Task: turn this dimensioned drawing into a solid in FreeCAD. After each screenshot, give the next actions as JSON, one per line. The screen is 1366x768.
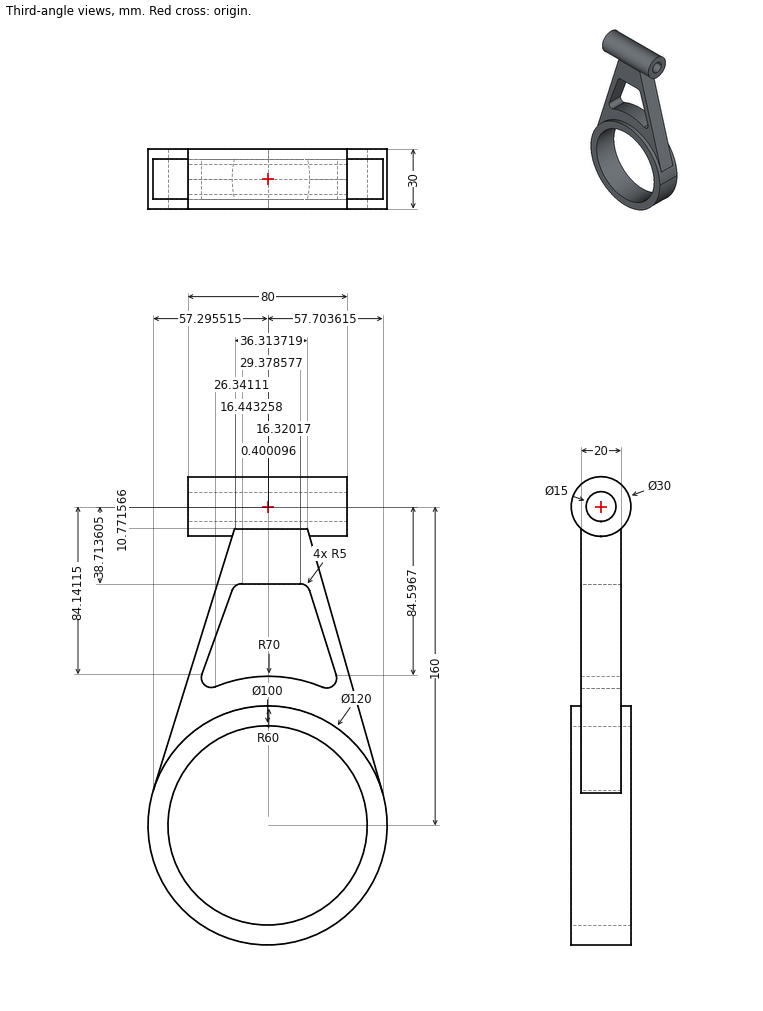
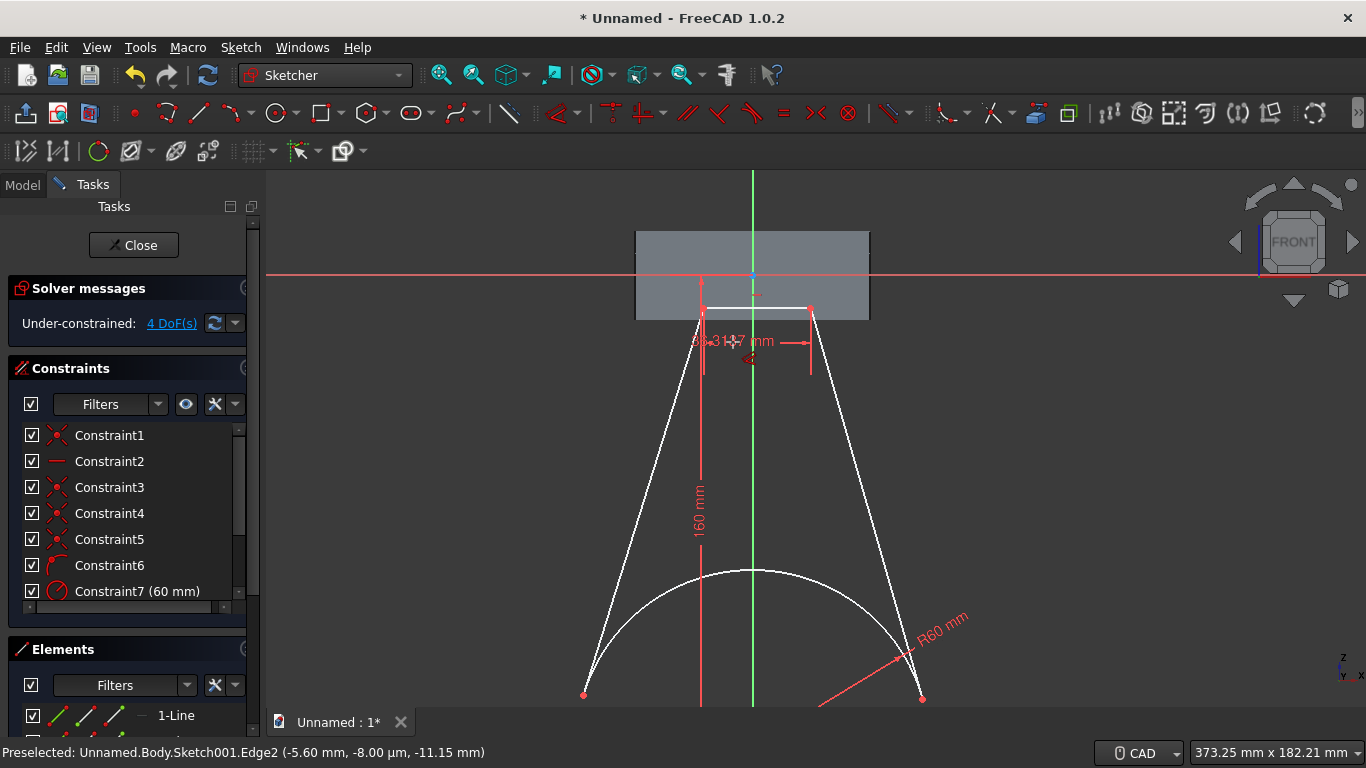
{"action": "scroll", "coordinate": [722, 220], "scroll_direction": "down", "scroll_amount": 1}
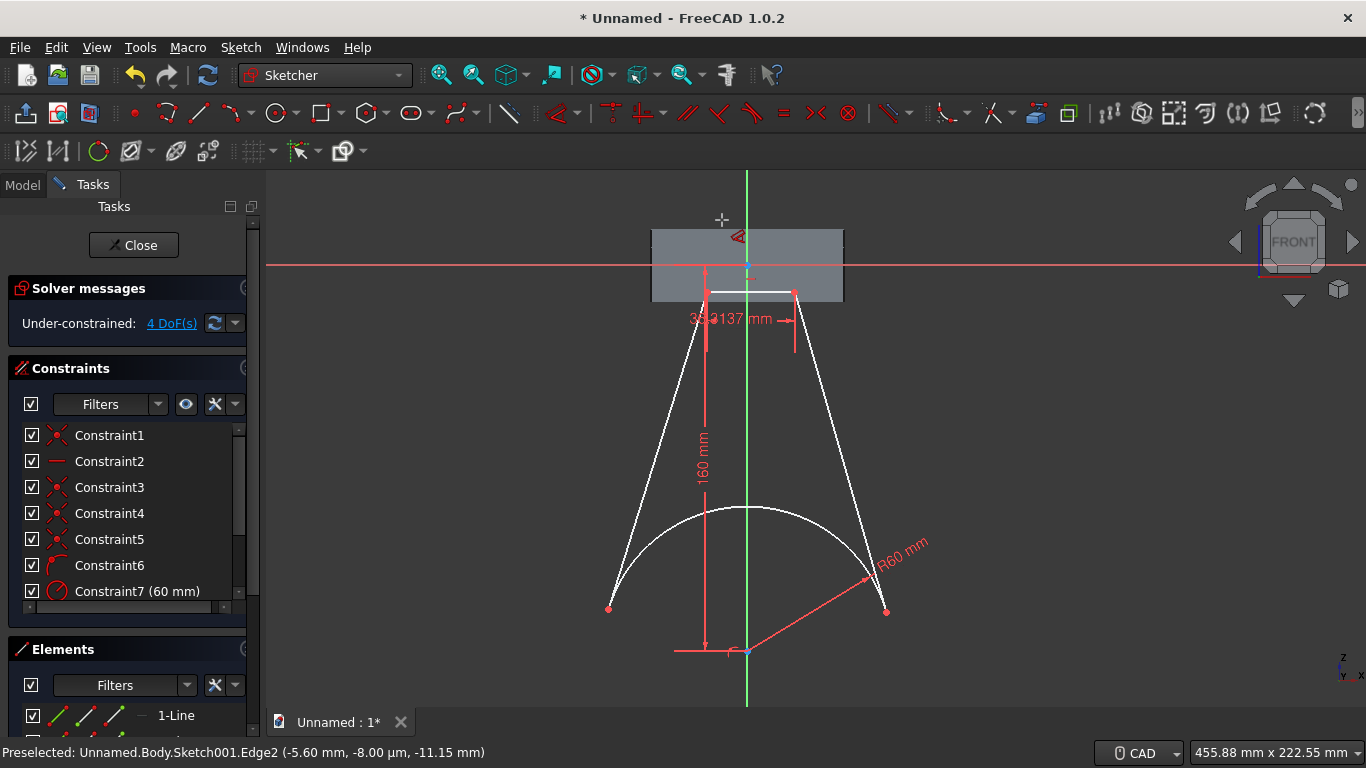
{"action": "left_click", "coordinate": [609, 609]}
{"action": "left_click", "coordinate": [678, 231]}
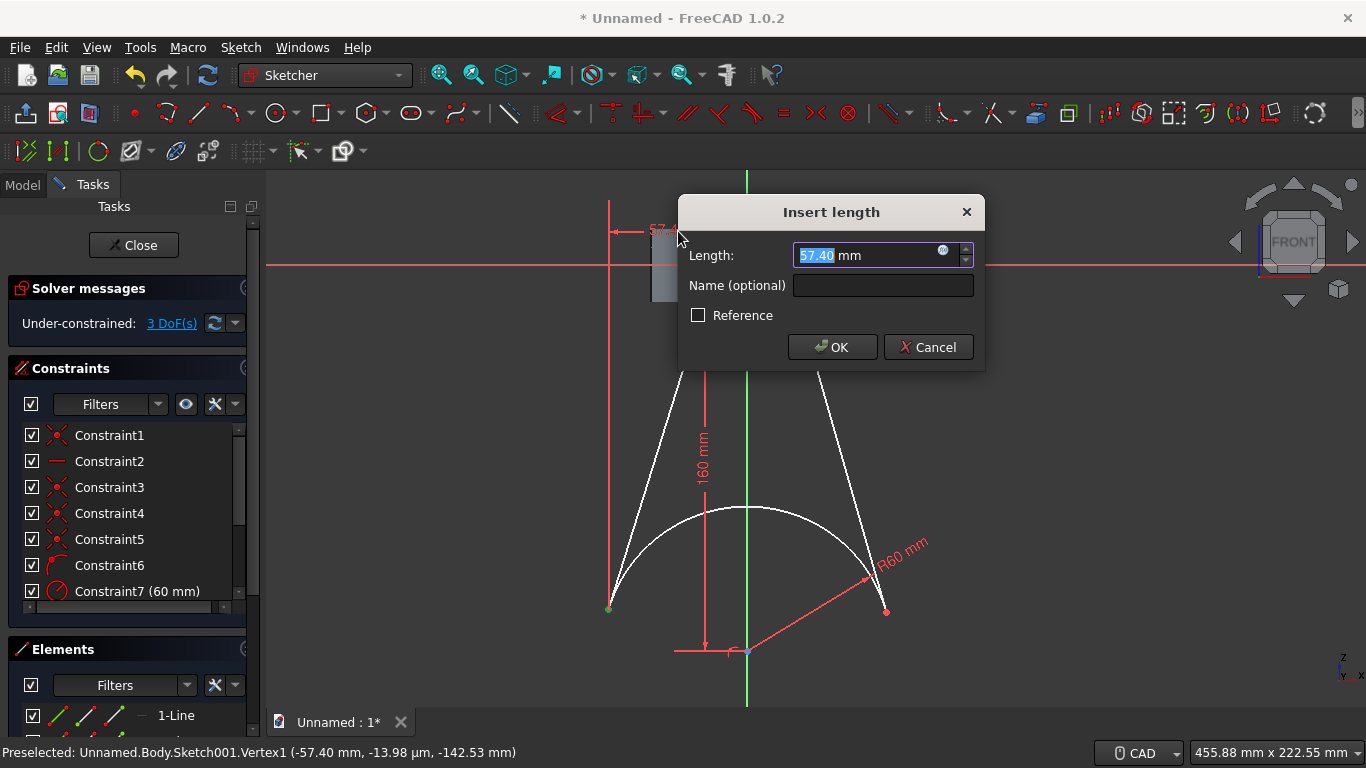
{"action": "type", "text": "57.295515"}
{"action": "key", "text": "Return"}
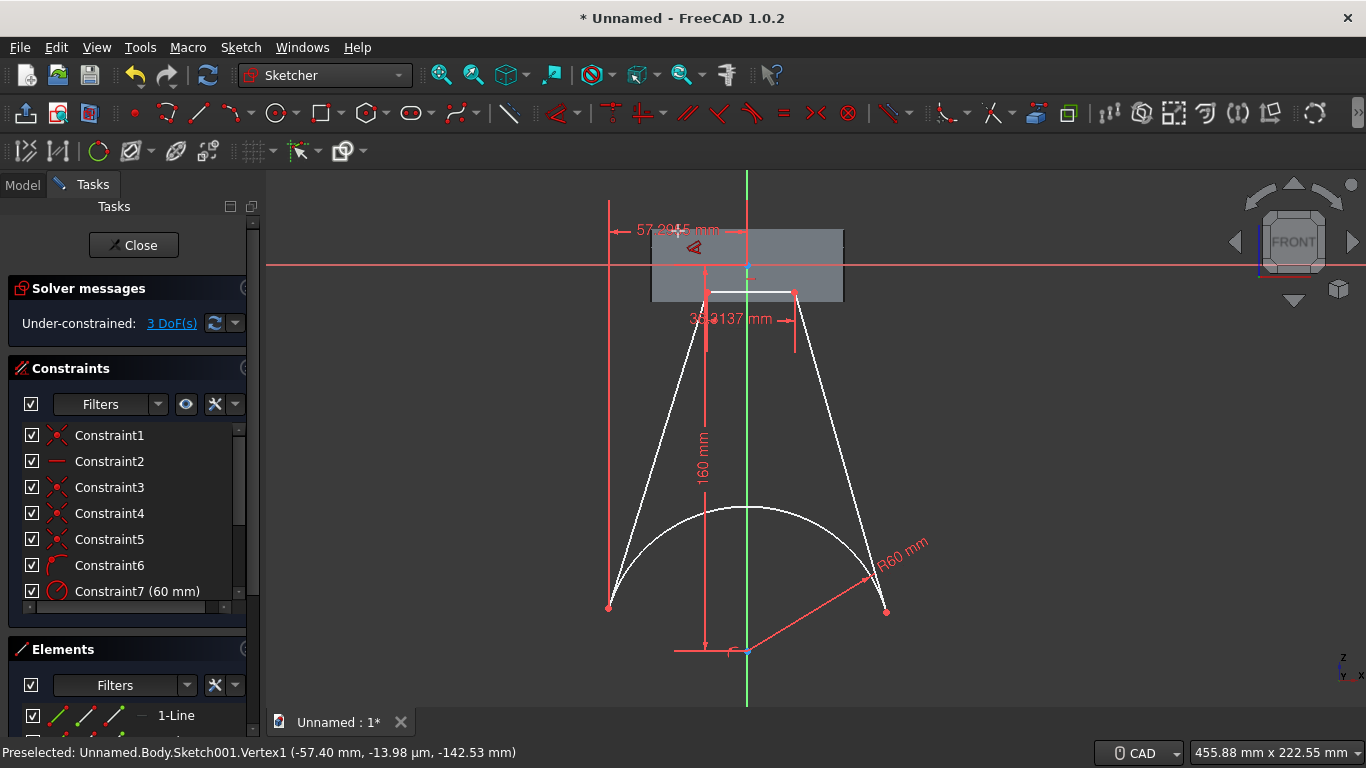
{"action": "left_click", "coordinate": [707, 292]}
{"action": "left_click", "coordinate": [727, 207]}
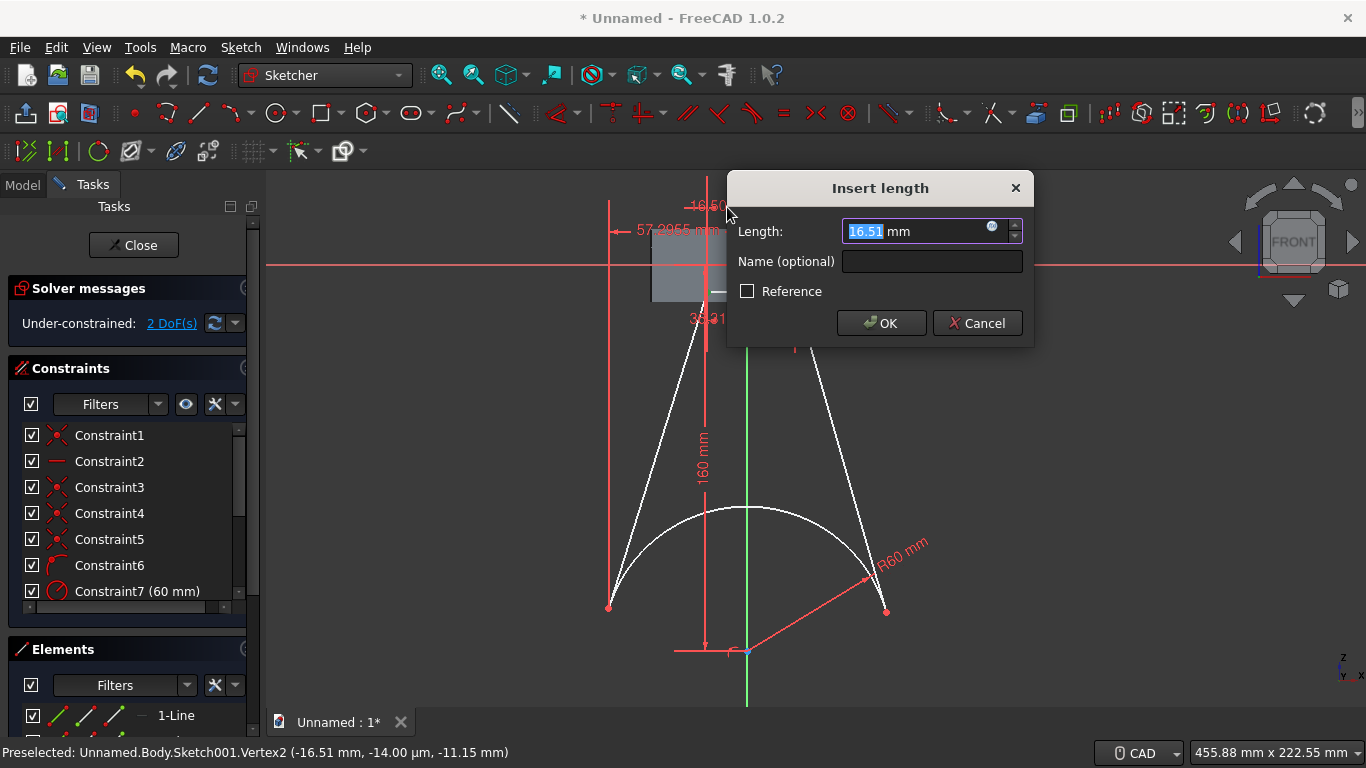
{"action": "type", "text": "16.443258"}
{"action": "key", "text": "Return"}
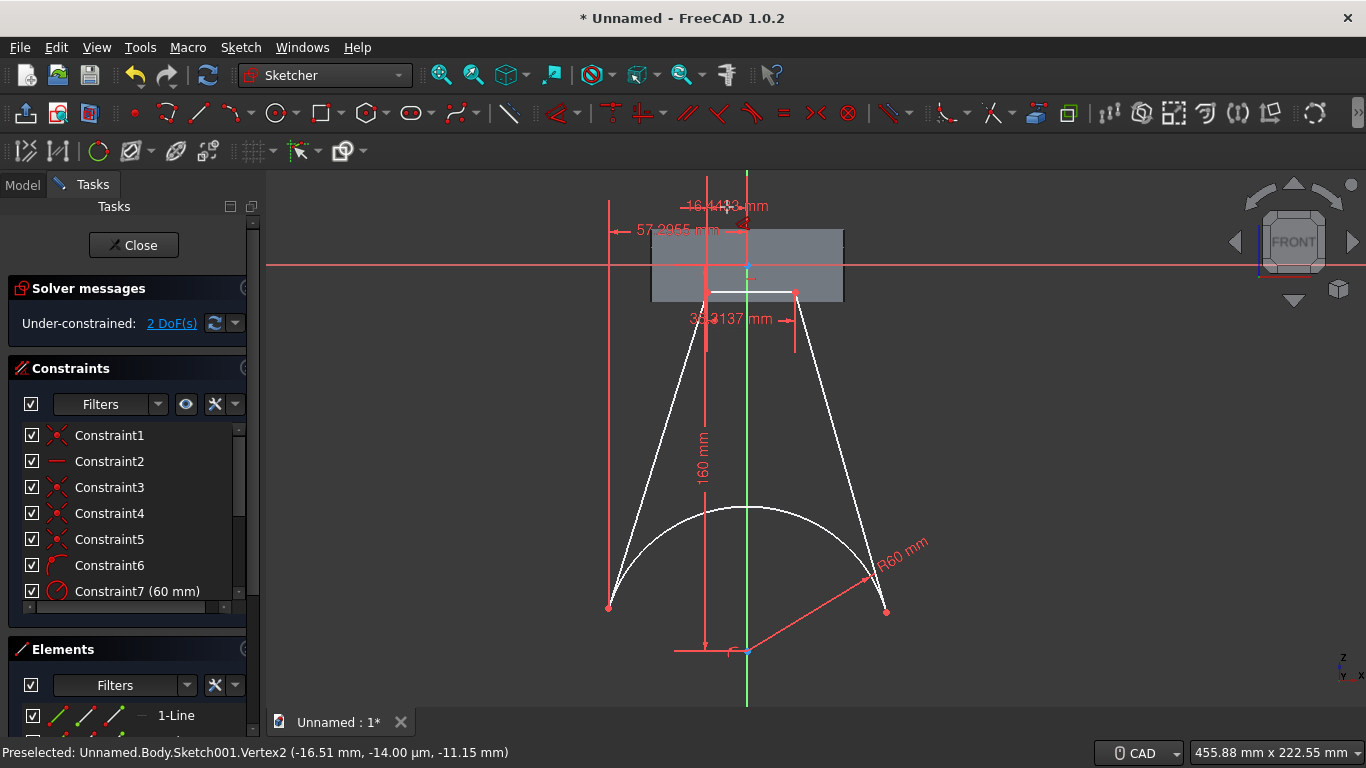
{"action": "scroll", "coordinate": [707, 292], "scroll_direction": "up", "scroll_amount": 3}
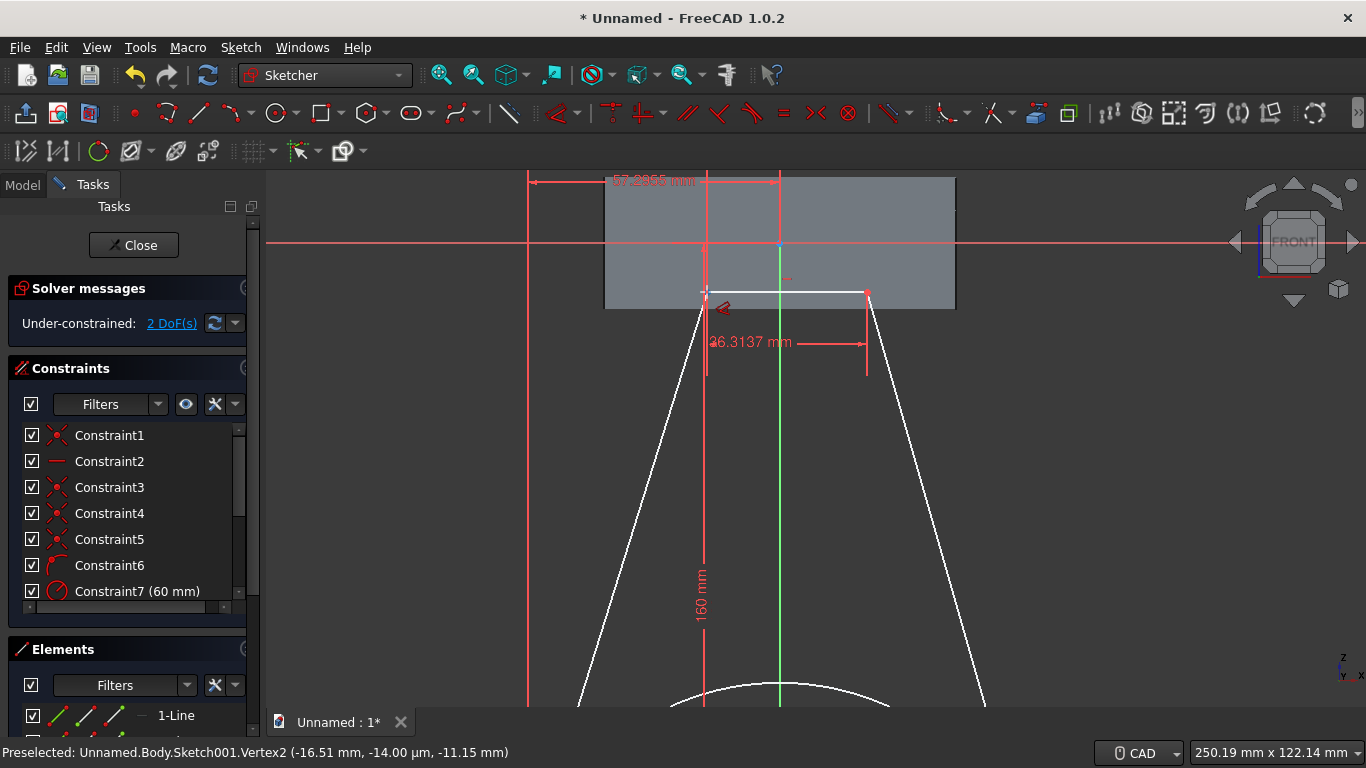
{"action": "left_click", "coordinate": [707, 292]}
{"action": "left_click", "coordinate": [673, 268]}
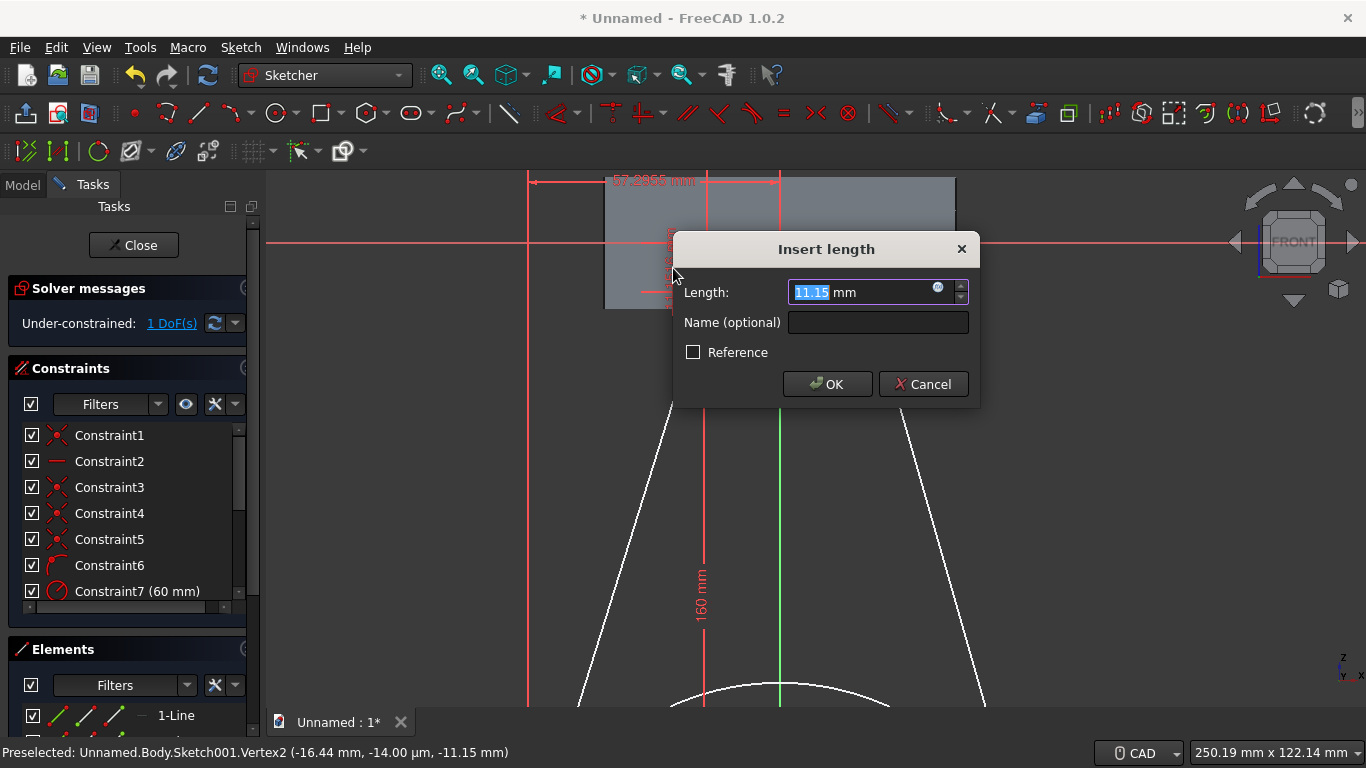
{"action": "type", "text": "10.771566"}
{"action": "key", "text": "Return"}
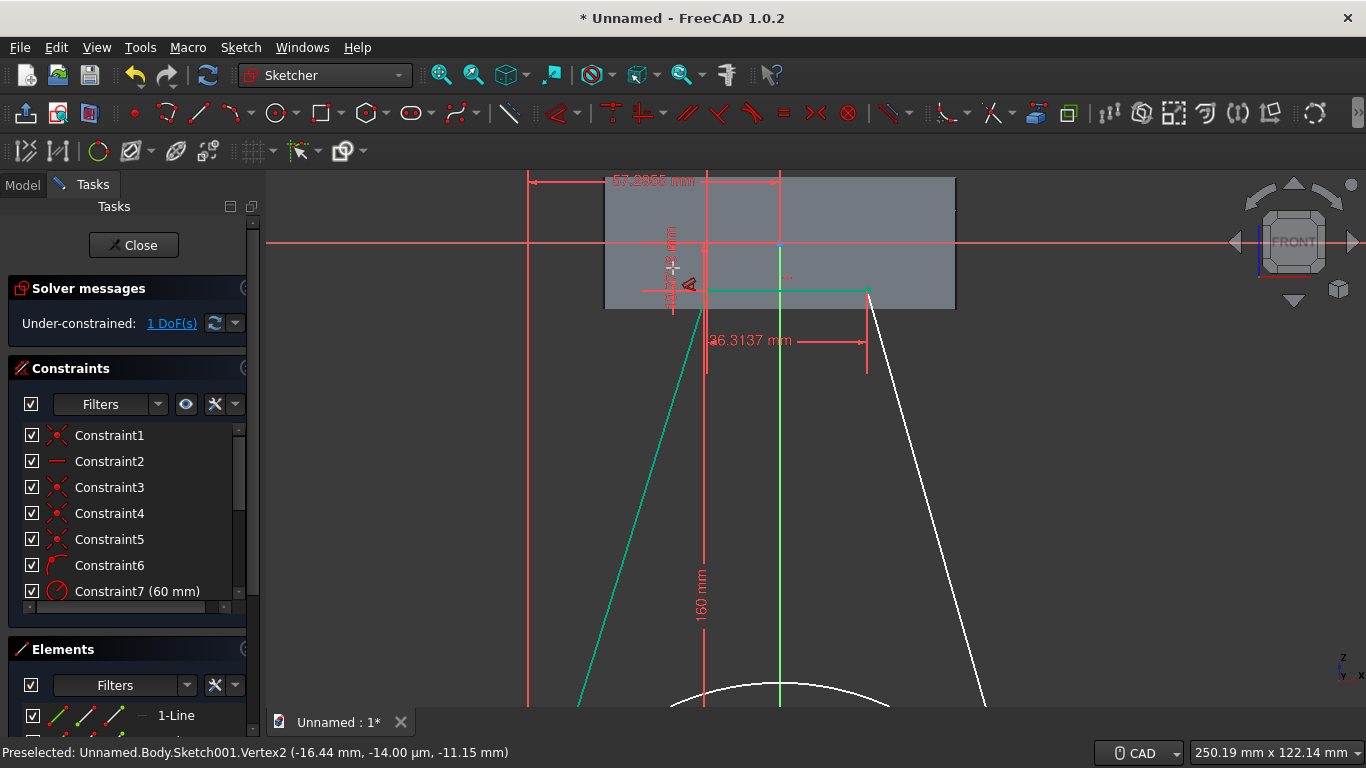
{"action": "scroll", "coordinate": [707, 292], "scroll_direction": "down", "scroll_amount": 3}